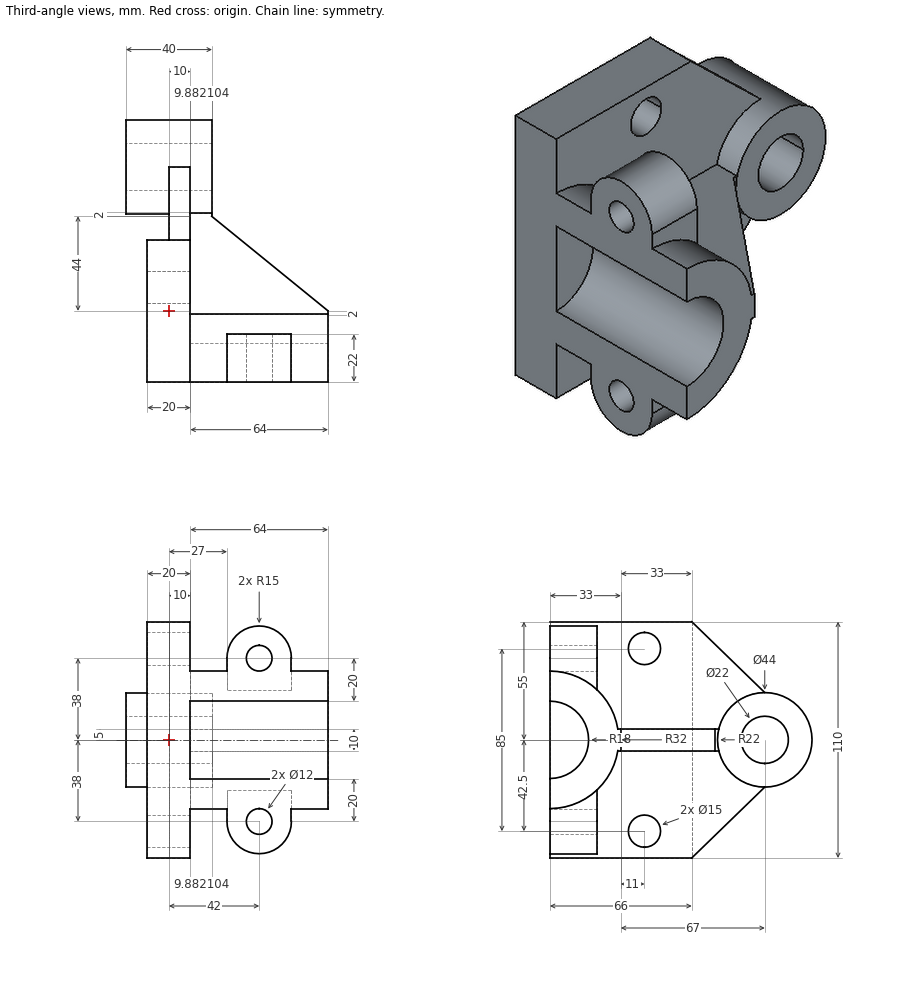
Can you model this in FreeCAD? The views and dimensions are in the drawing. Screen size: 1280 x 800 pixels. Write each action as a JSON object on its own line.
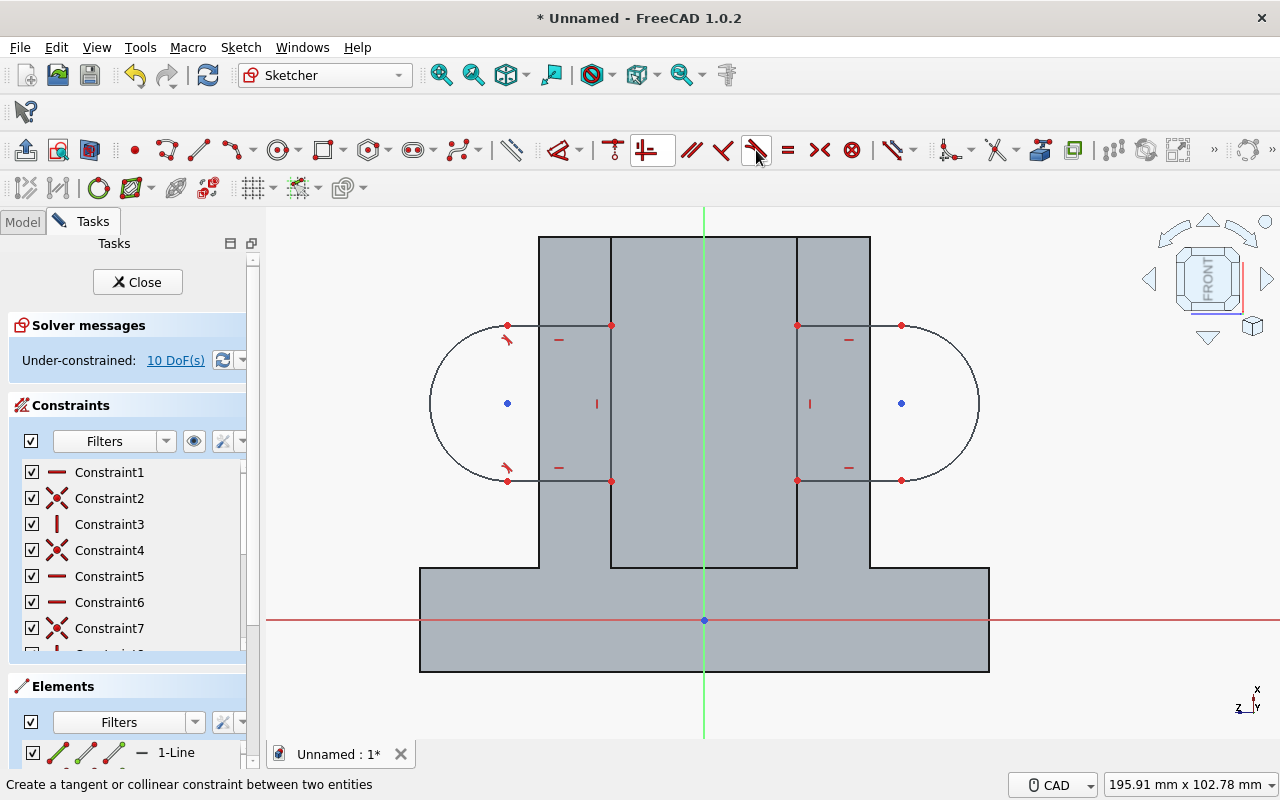
{"action": "left_click", "coordinate": [870, 326]}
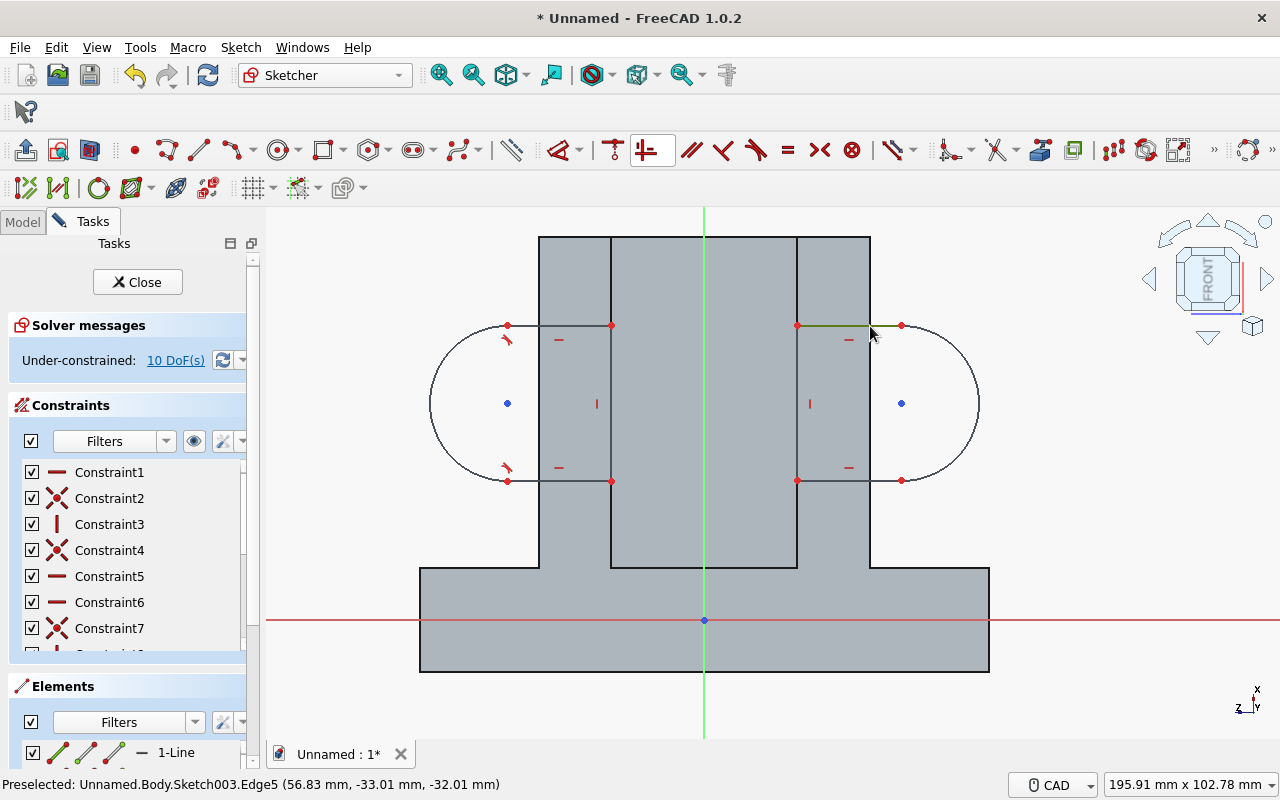
{"action": "left_click", "coordinate": [964, 449]}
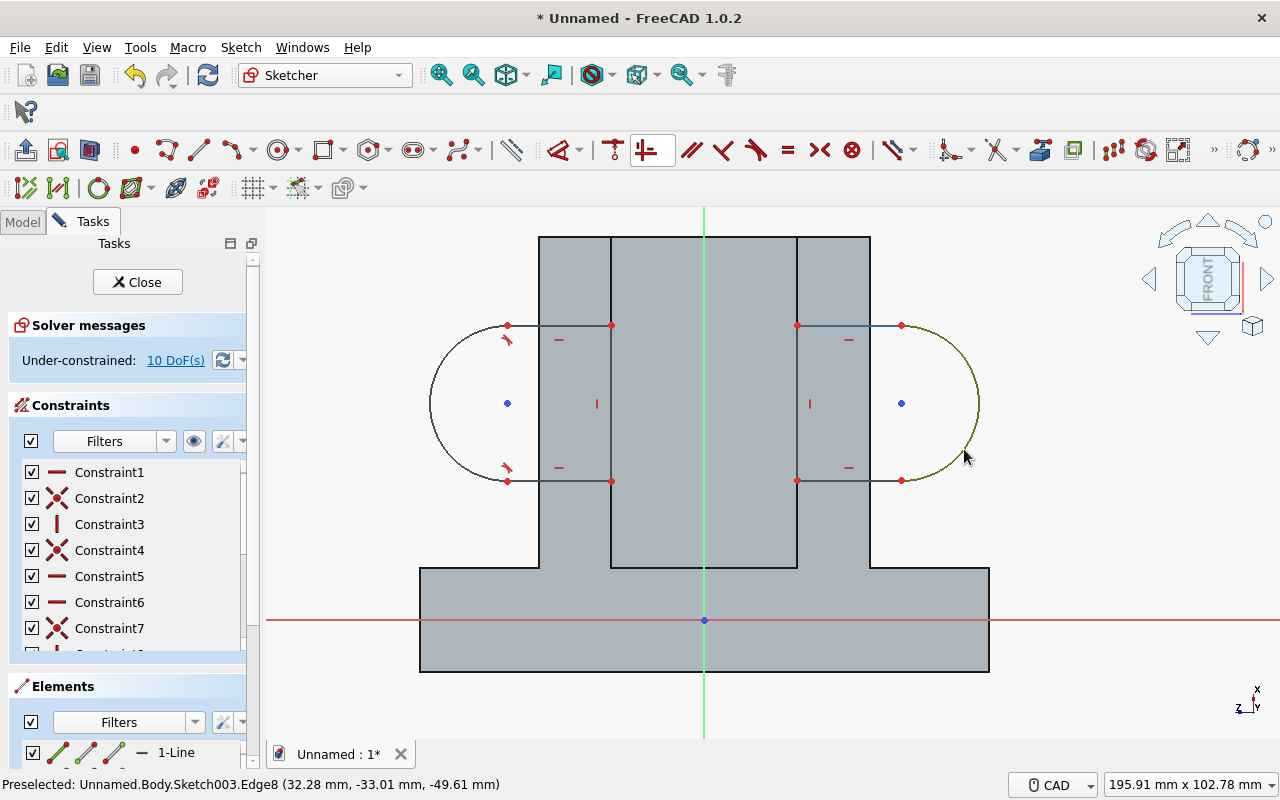
{"action": "left_click", "coordinate": [756, 150]}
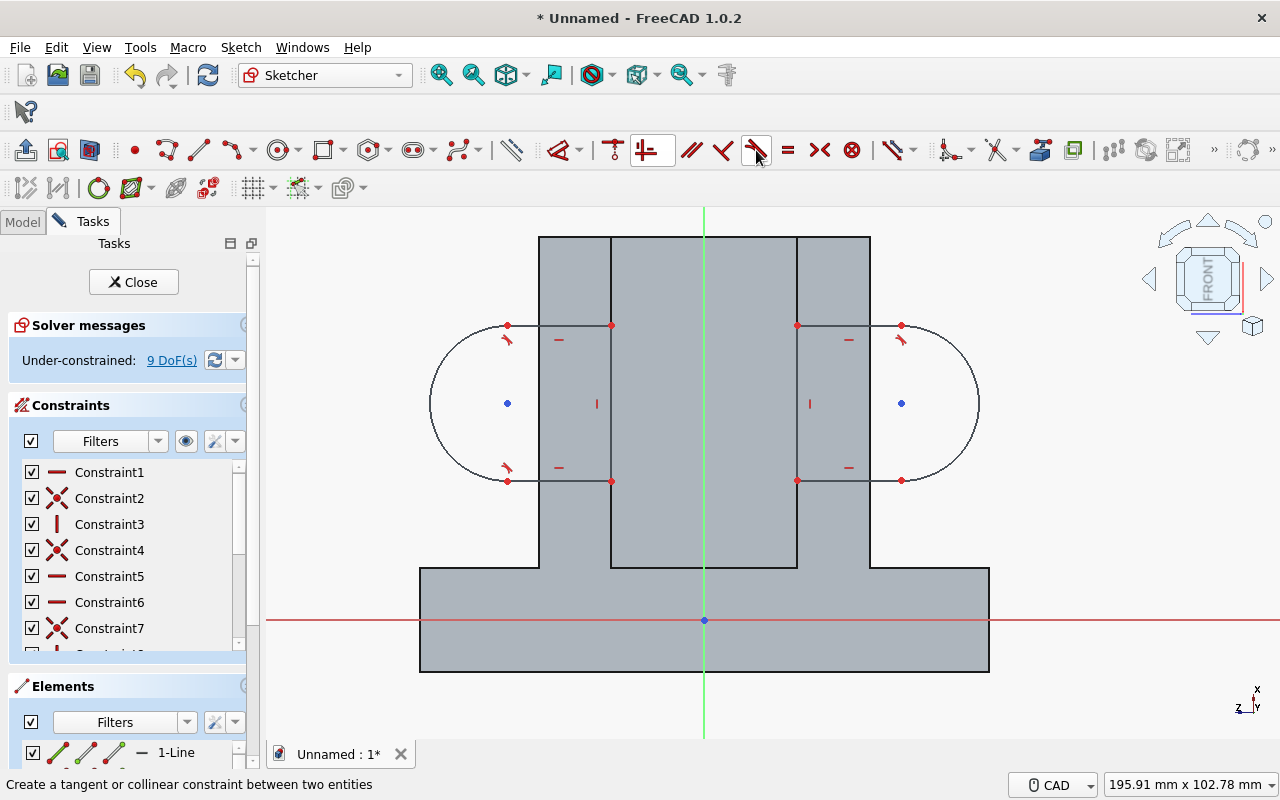
{"action": "left_click", "coordinate": [828, 481]}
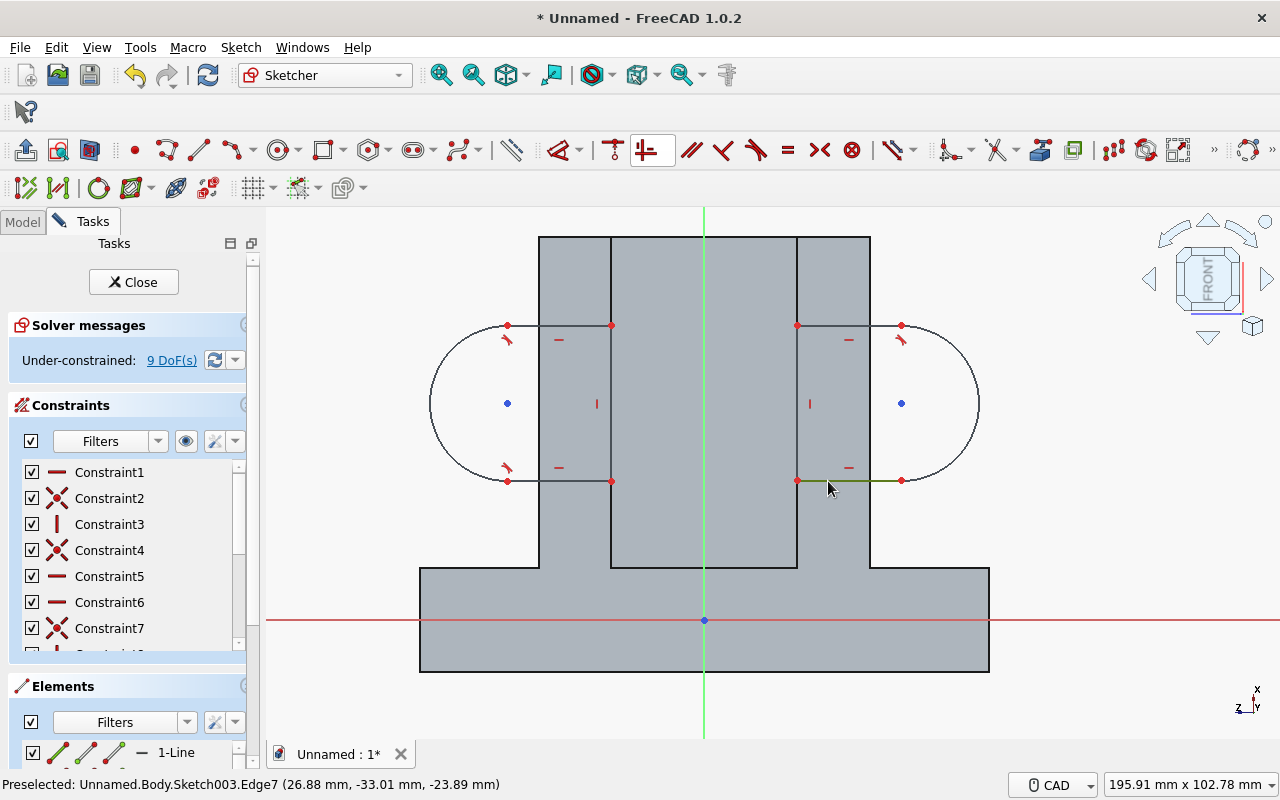
{"action": "left_click", "coordinate": [964, 449]}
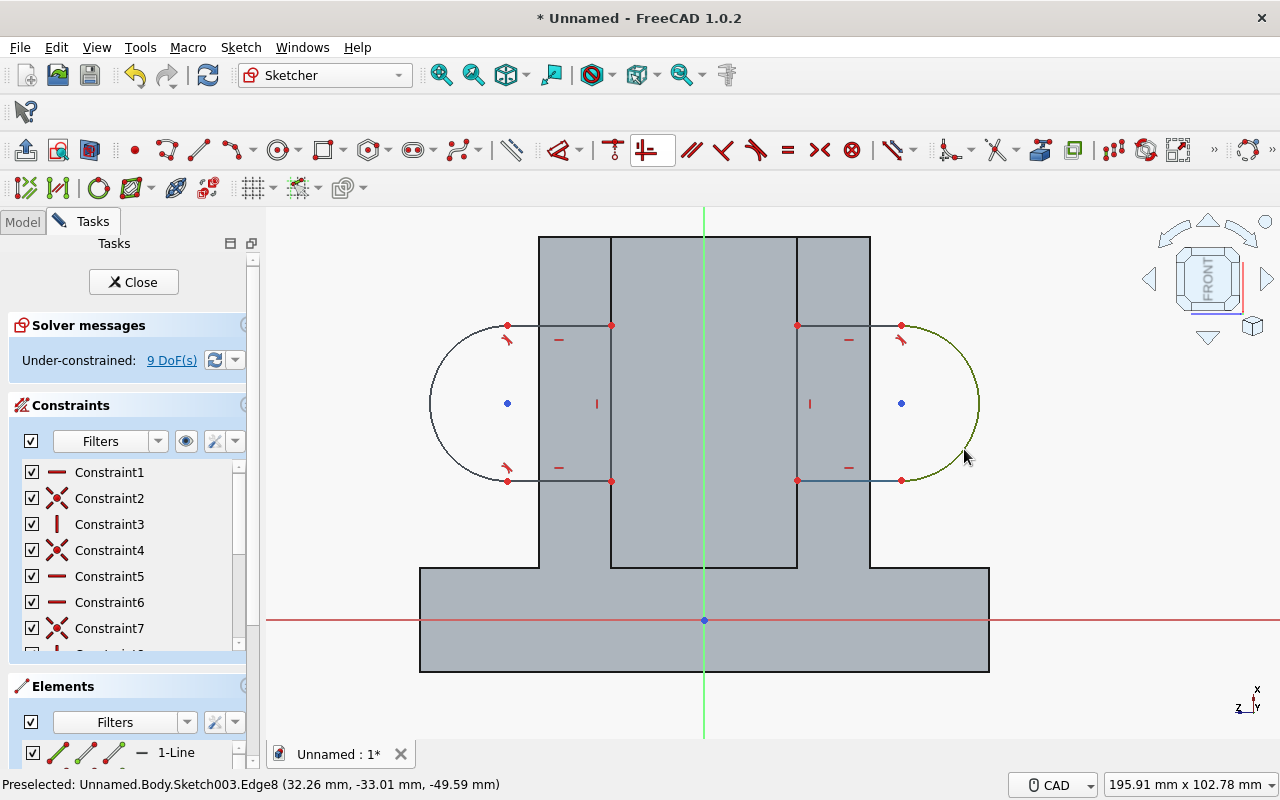
{"action": "left_click", "coordinate": [756, 150]}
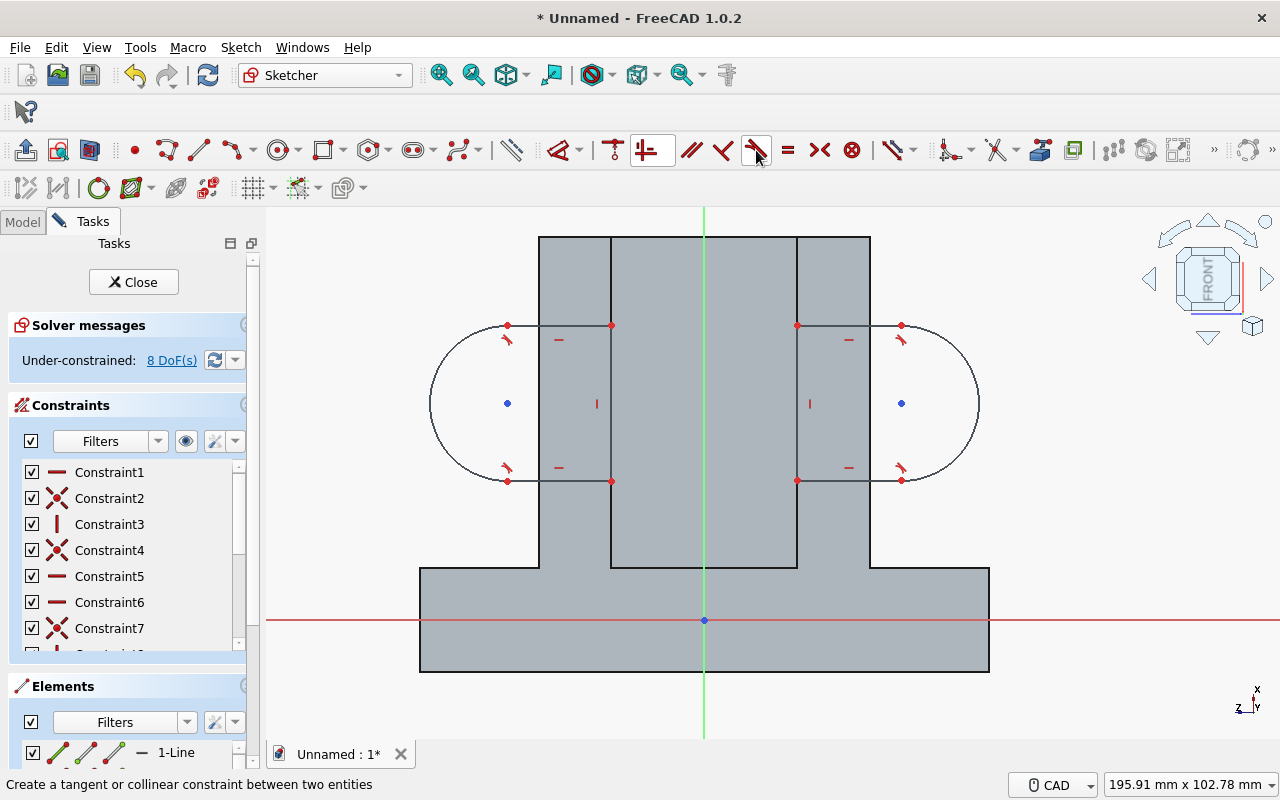
{"action": "left_click", "coordinate": [445, 358]}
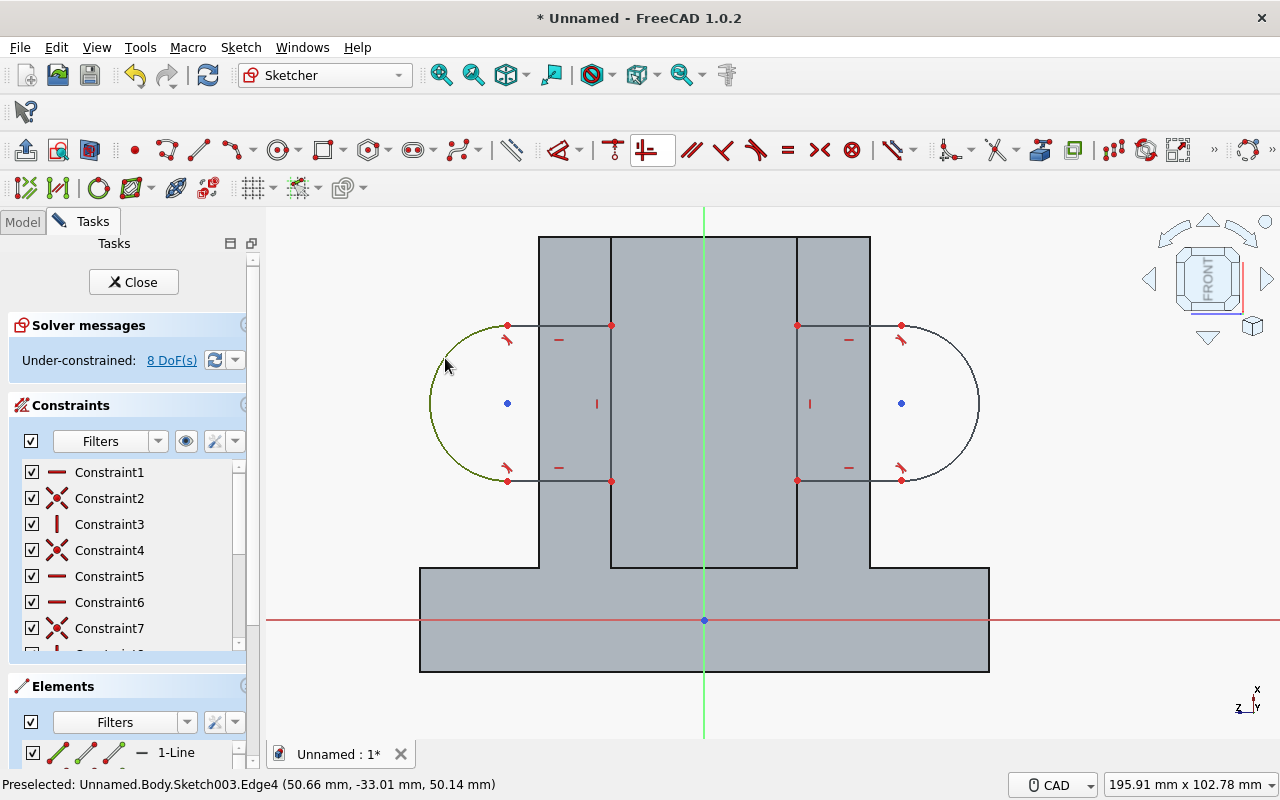
{"action": "left_click", "coordinate": [964, 449]}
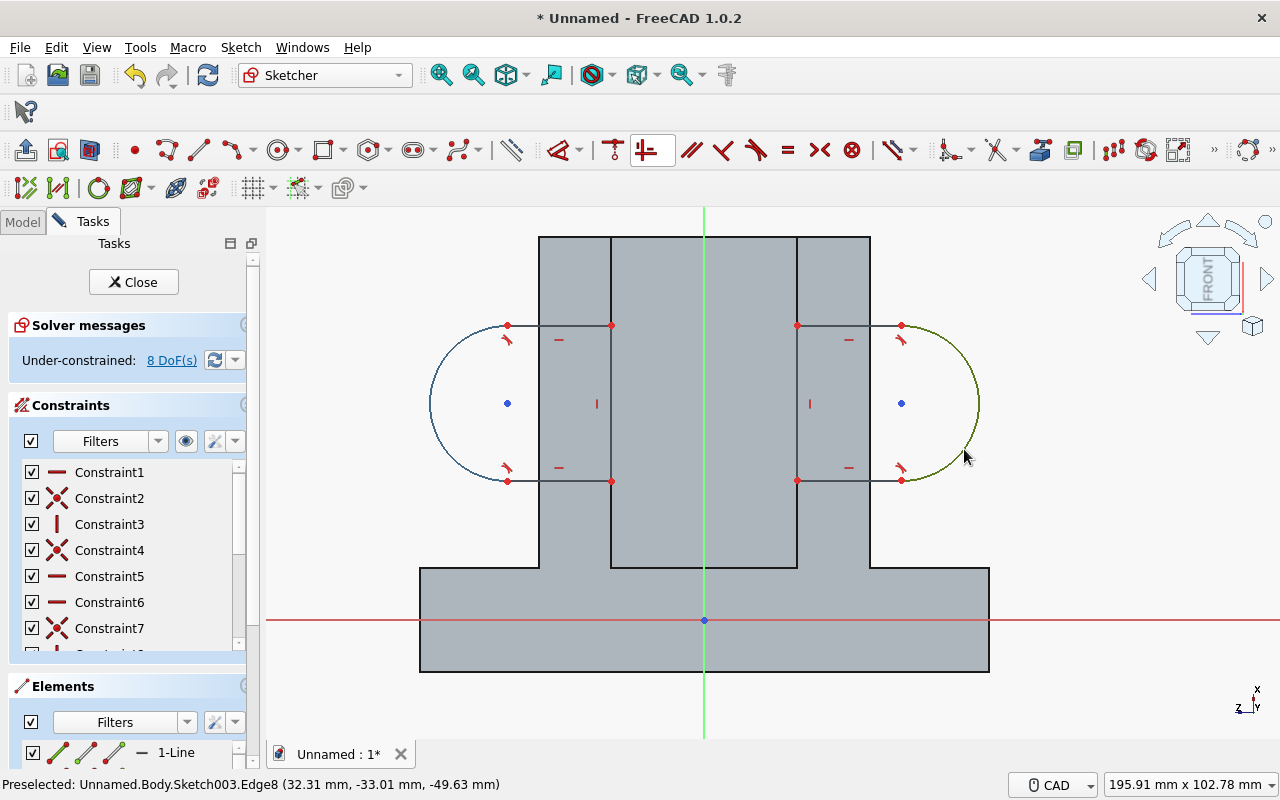
{"action": "left_click", "coordinate": [788, 150]}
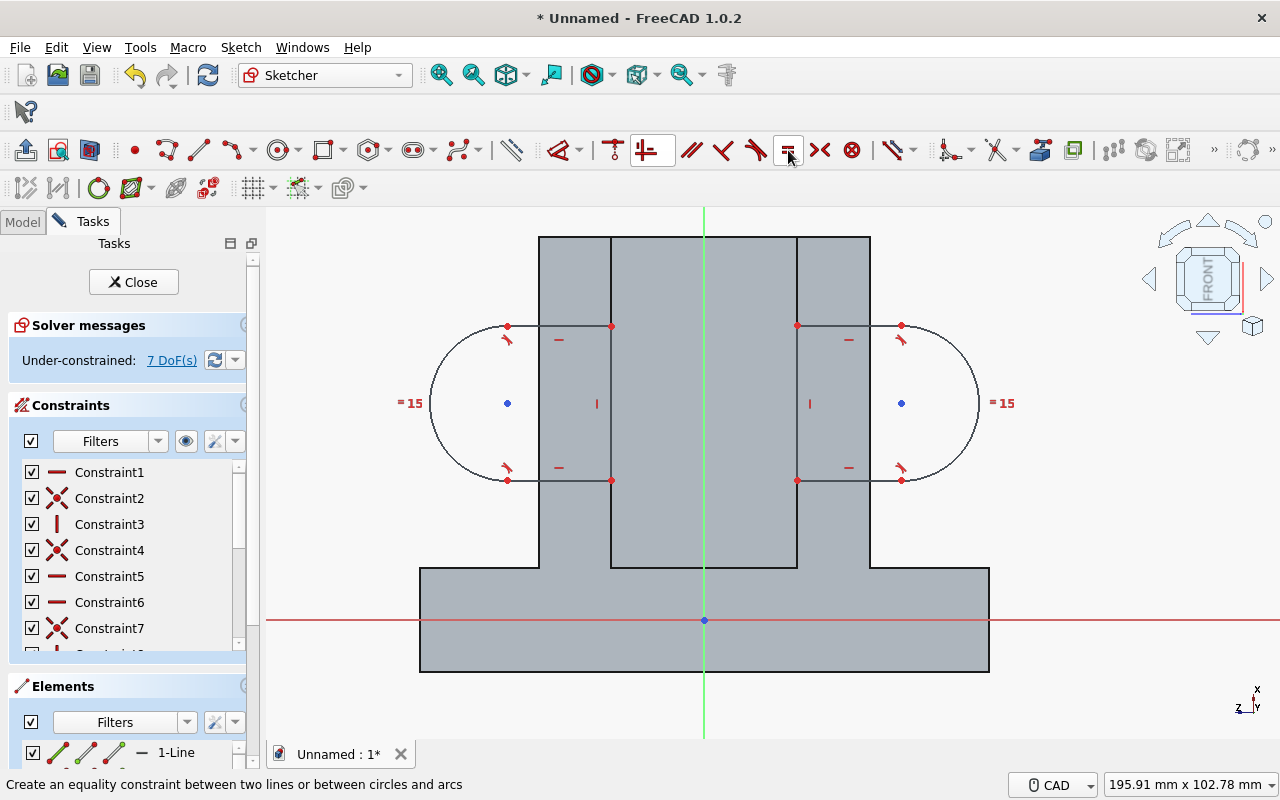
{"action": "left_click", "coordinate": [508, 404]}